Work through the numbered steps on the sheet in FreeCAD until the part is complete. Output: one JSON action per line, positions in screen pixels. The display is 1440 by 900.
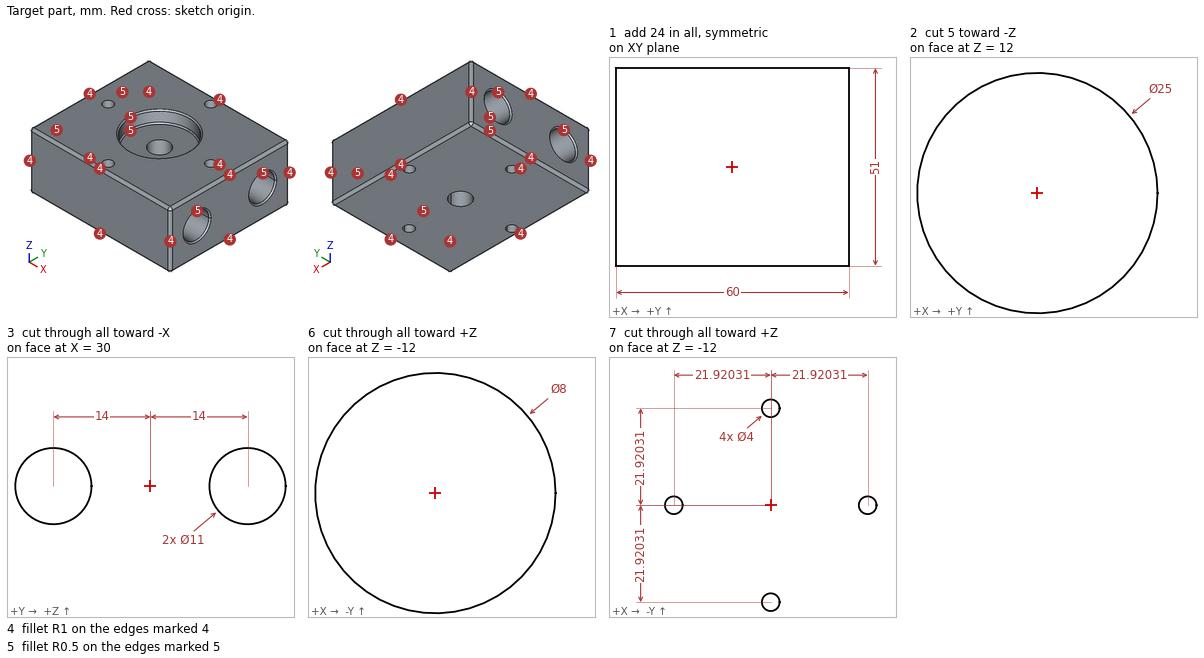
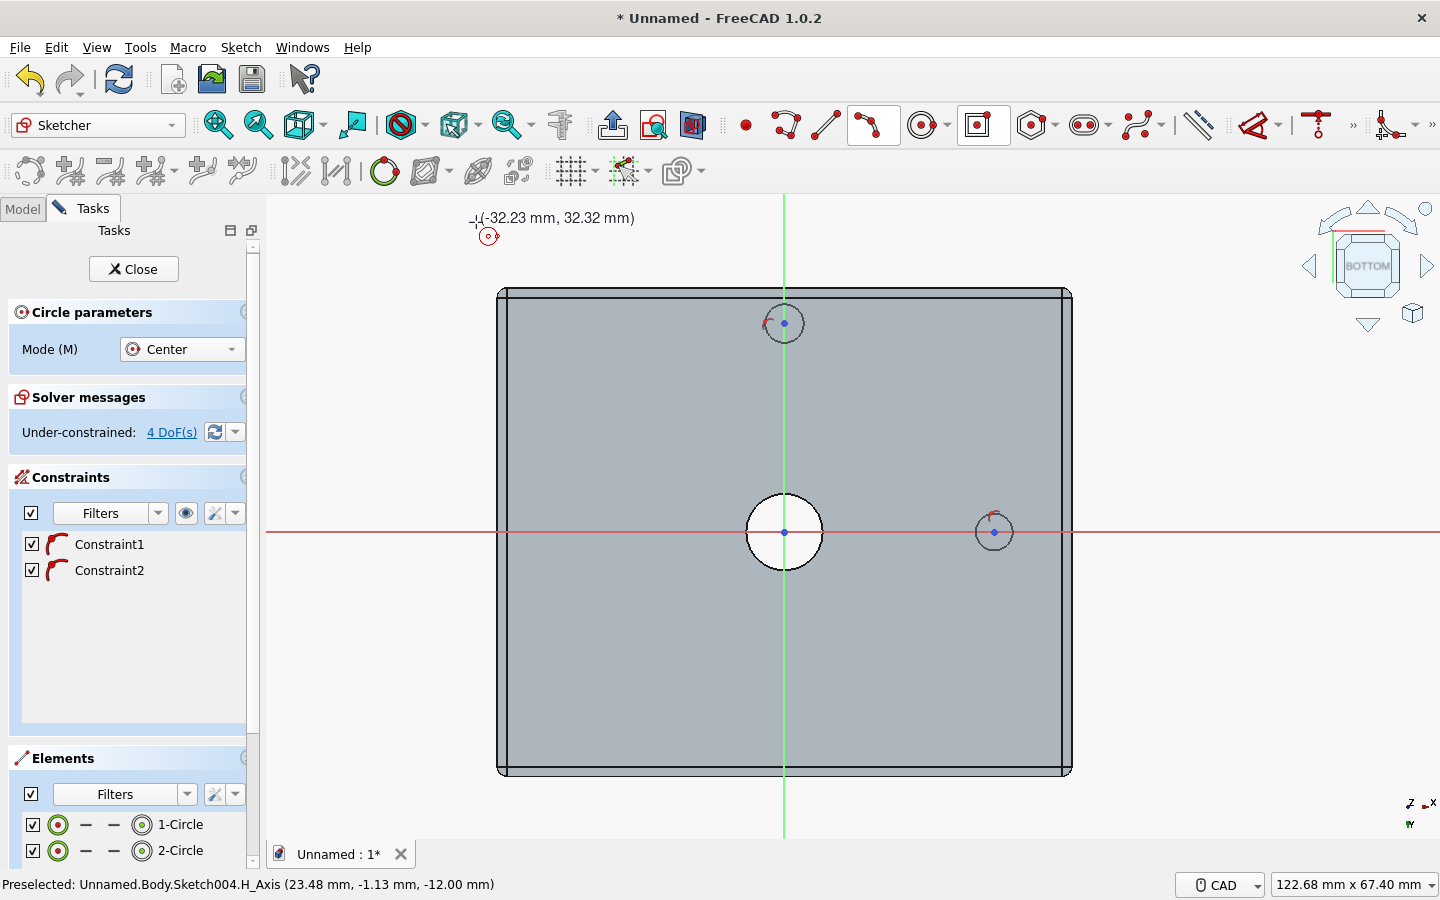
{"action": "left_click", "coordinate": [784, 742]}
{"action": "left_click", "coordinate": [802, 735]}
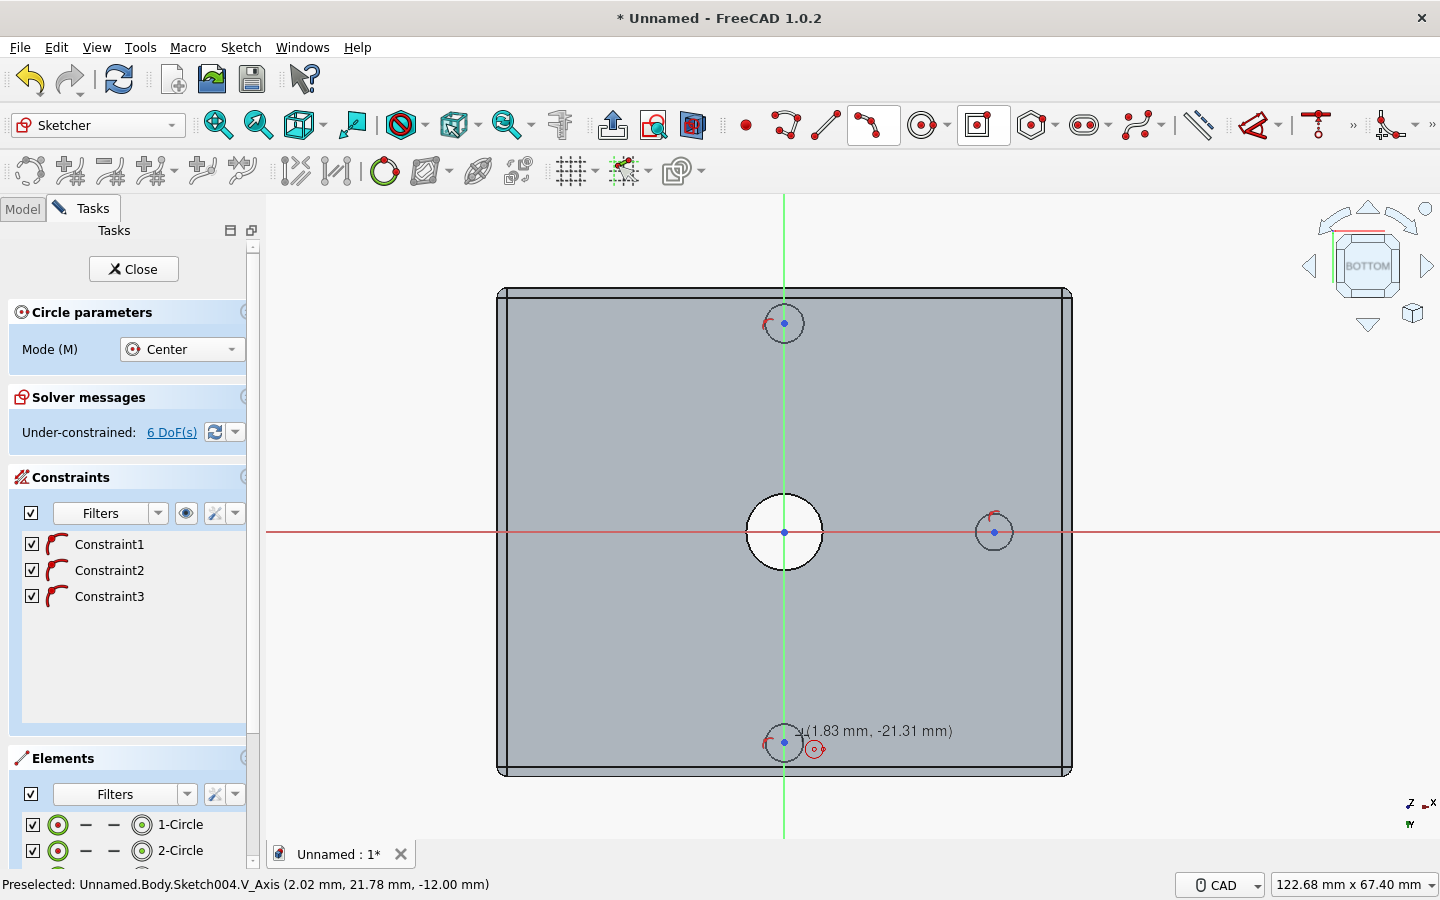
{"action": "left_click", "coordinate": [575, 532]}
{"action": "left_click", "coordinate": [581, 514]}
{"action": "key", "text": "Escape"}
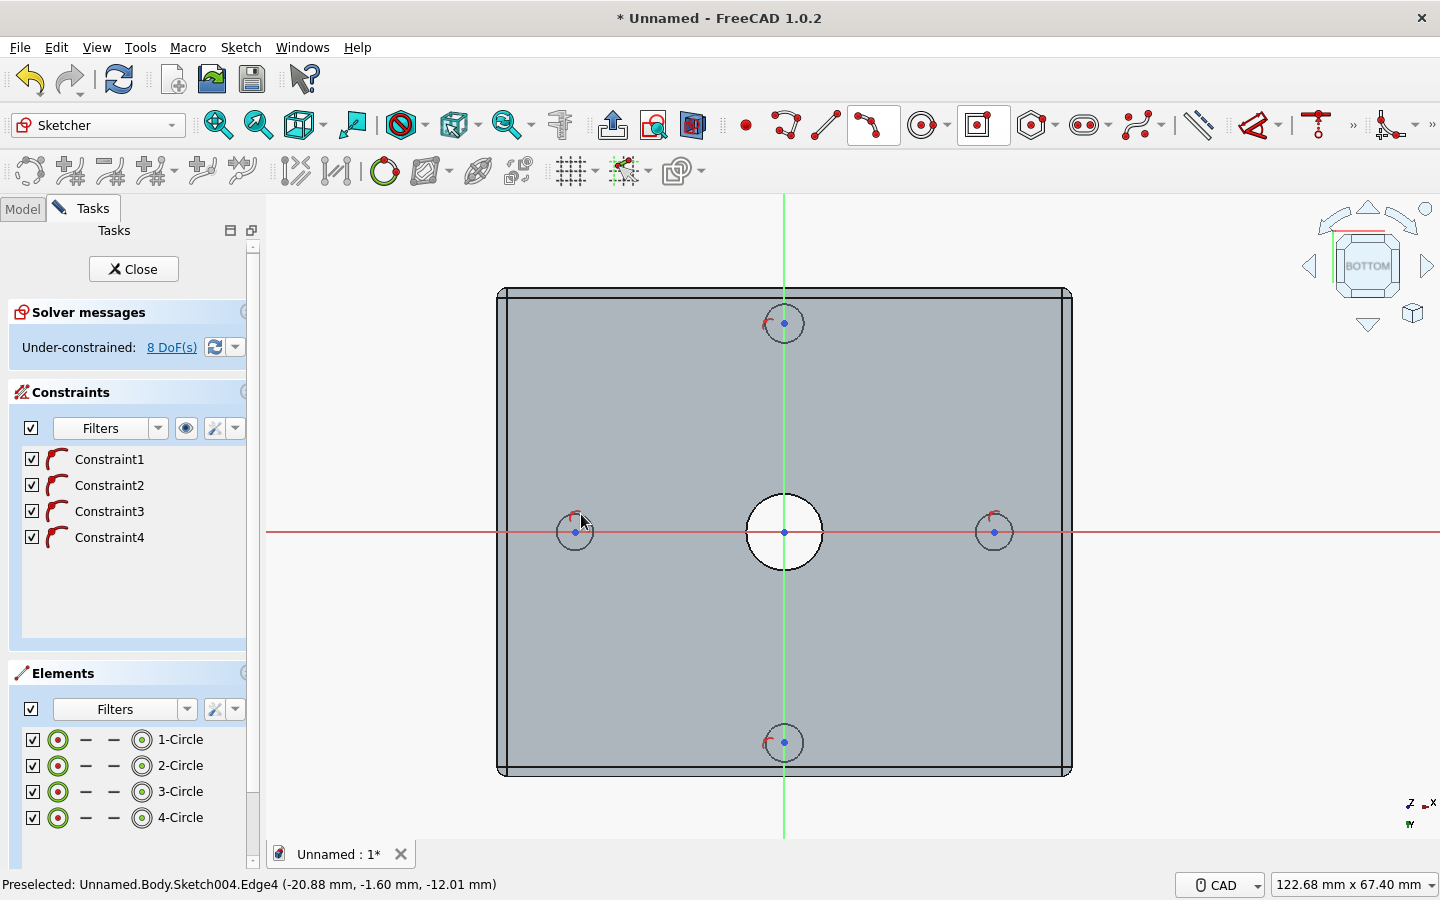
{"action": "left_click", "coordinate": [798, 310]}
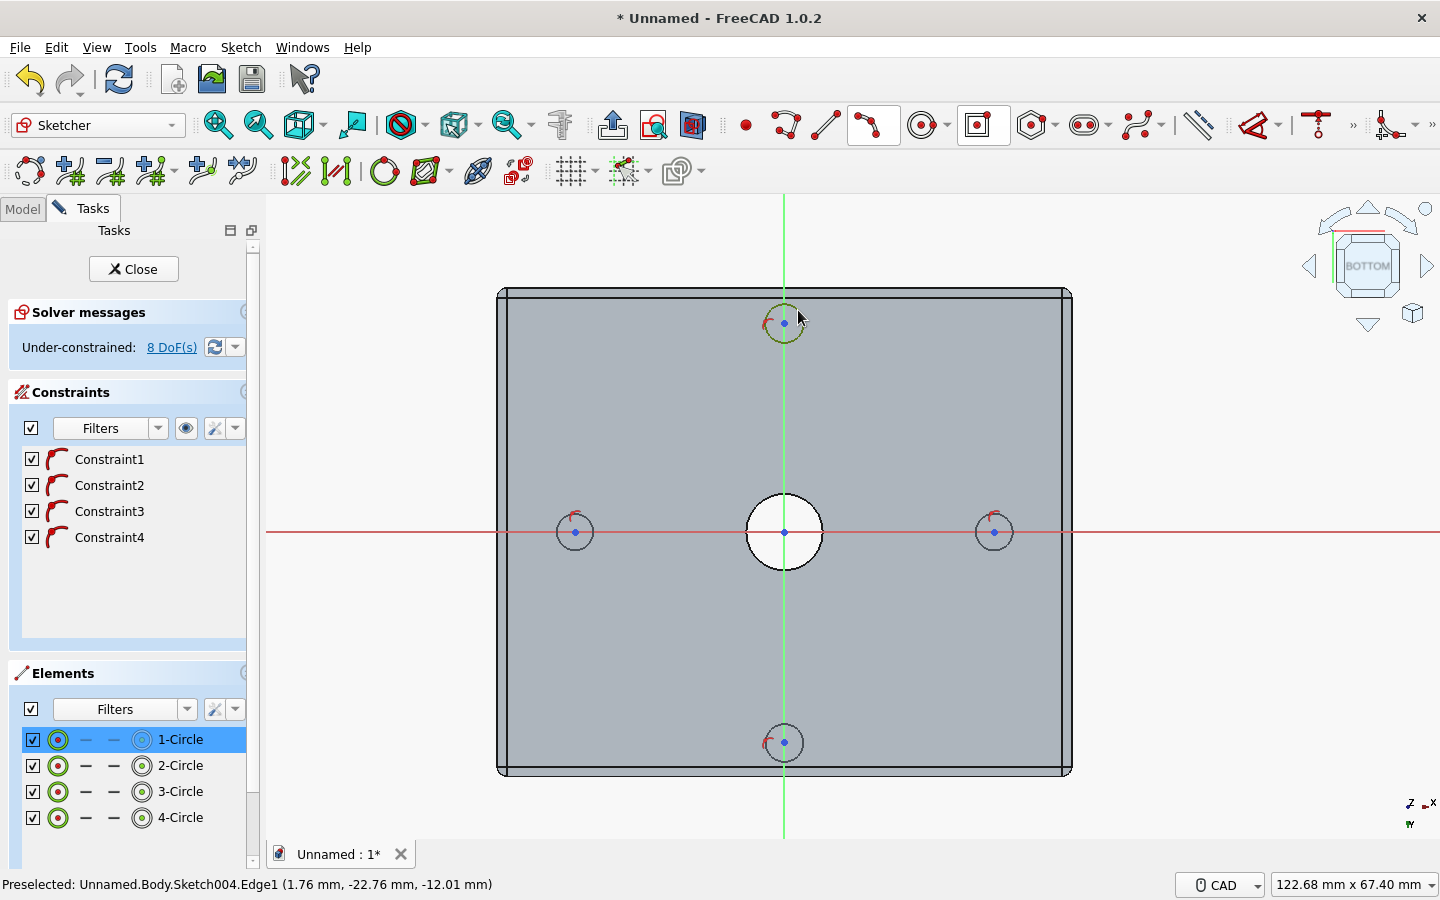
{"action": "left_click", "coordinate": [1007, 519]}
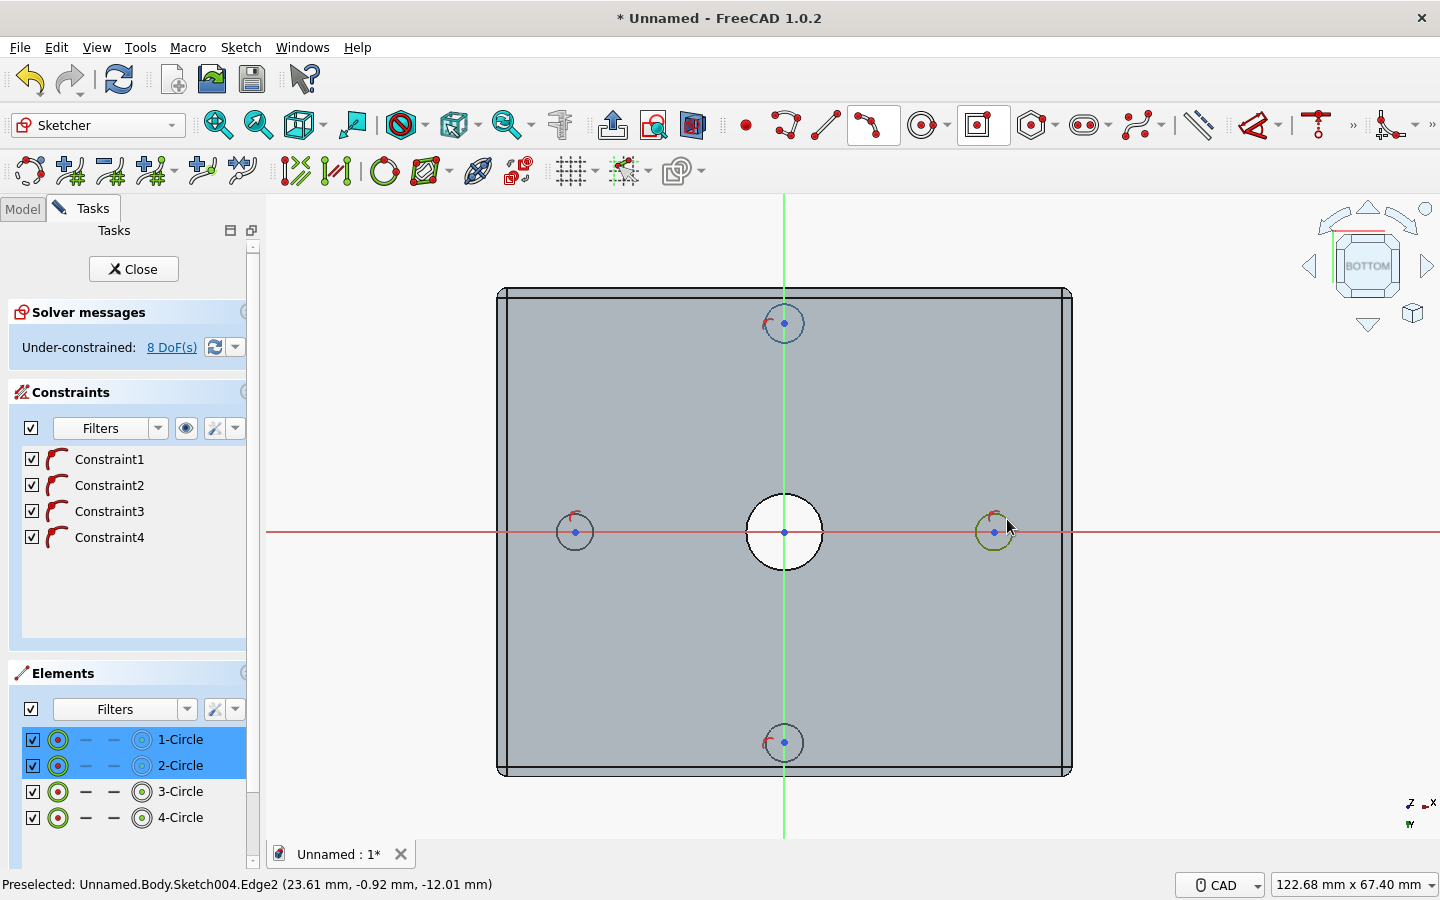
{"action": "left_click", "coordinate": [798, 730]}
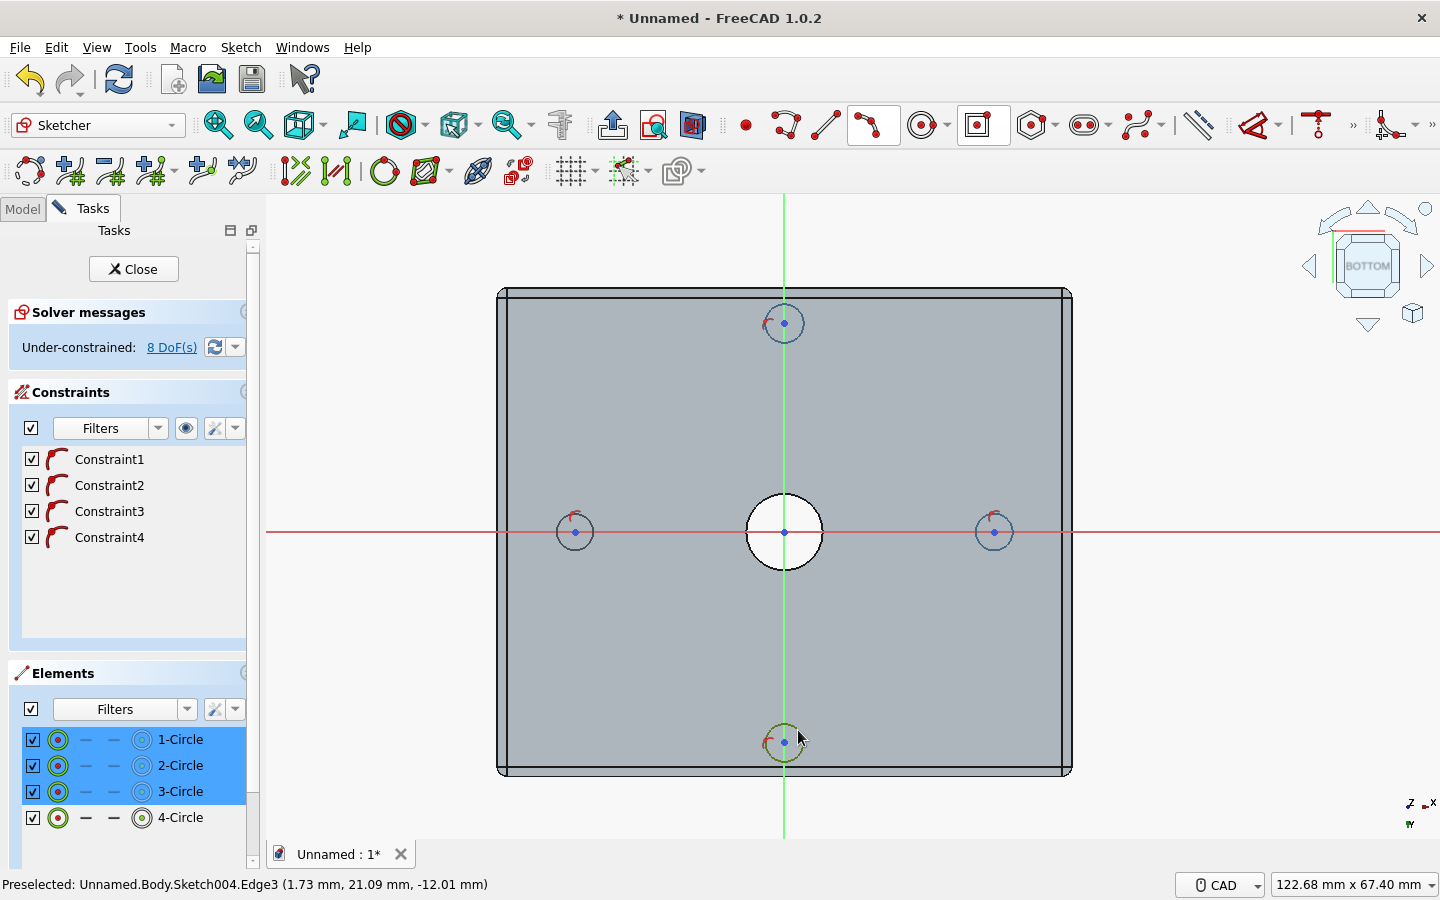
{"action": "left_click", "coordinate": [588, 519]}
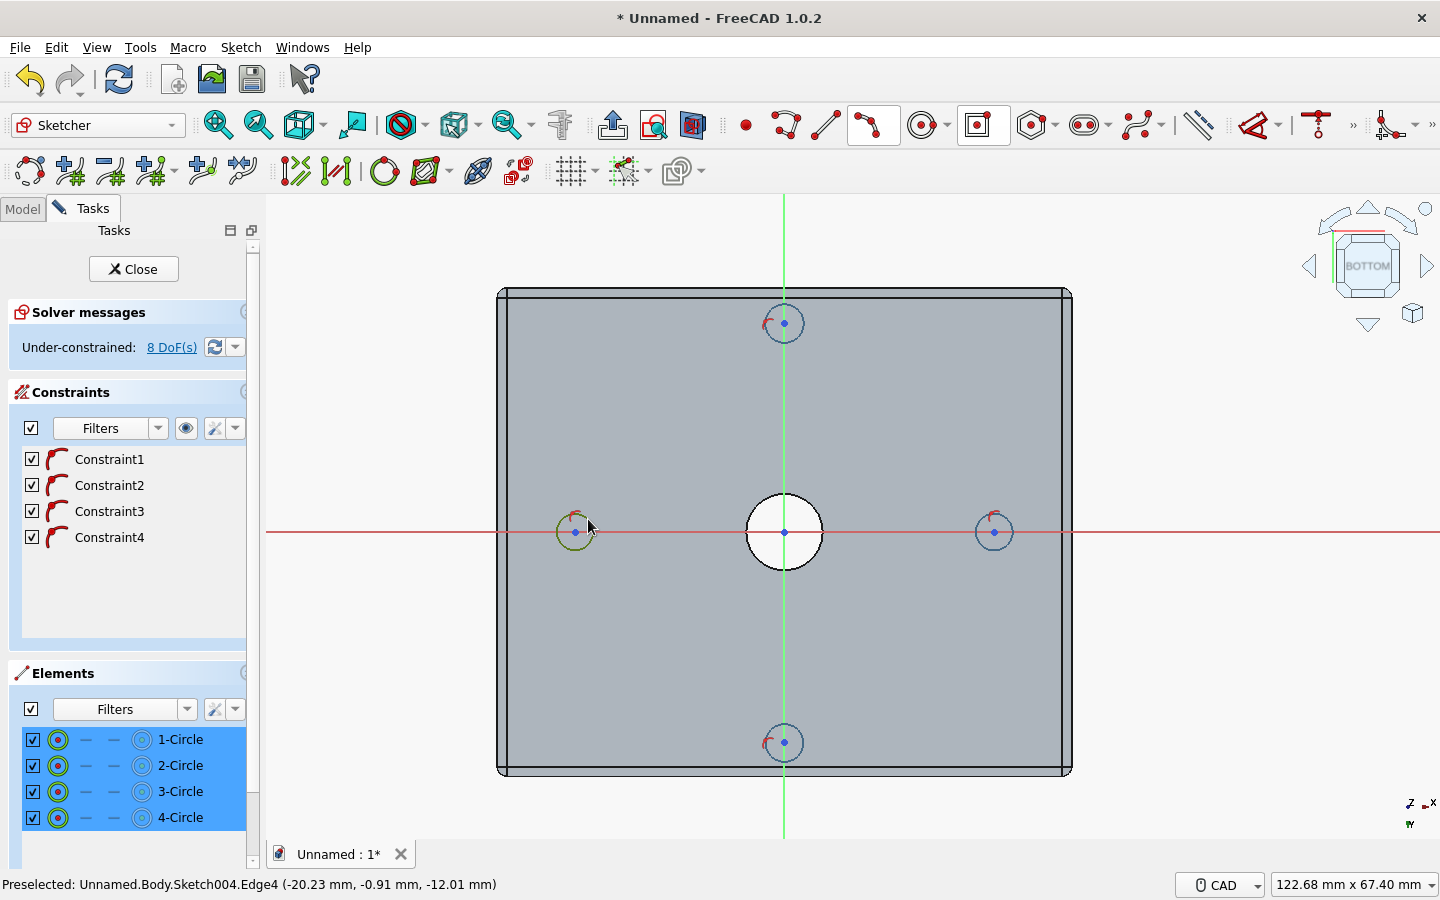
{"action": "key", "text": "e"}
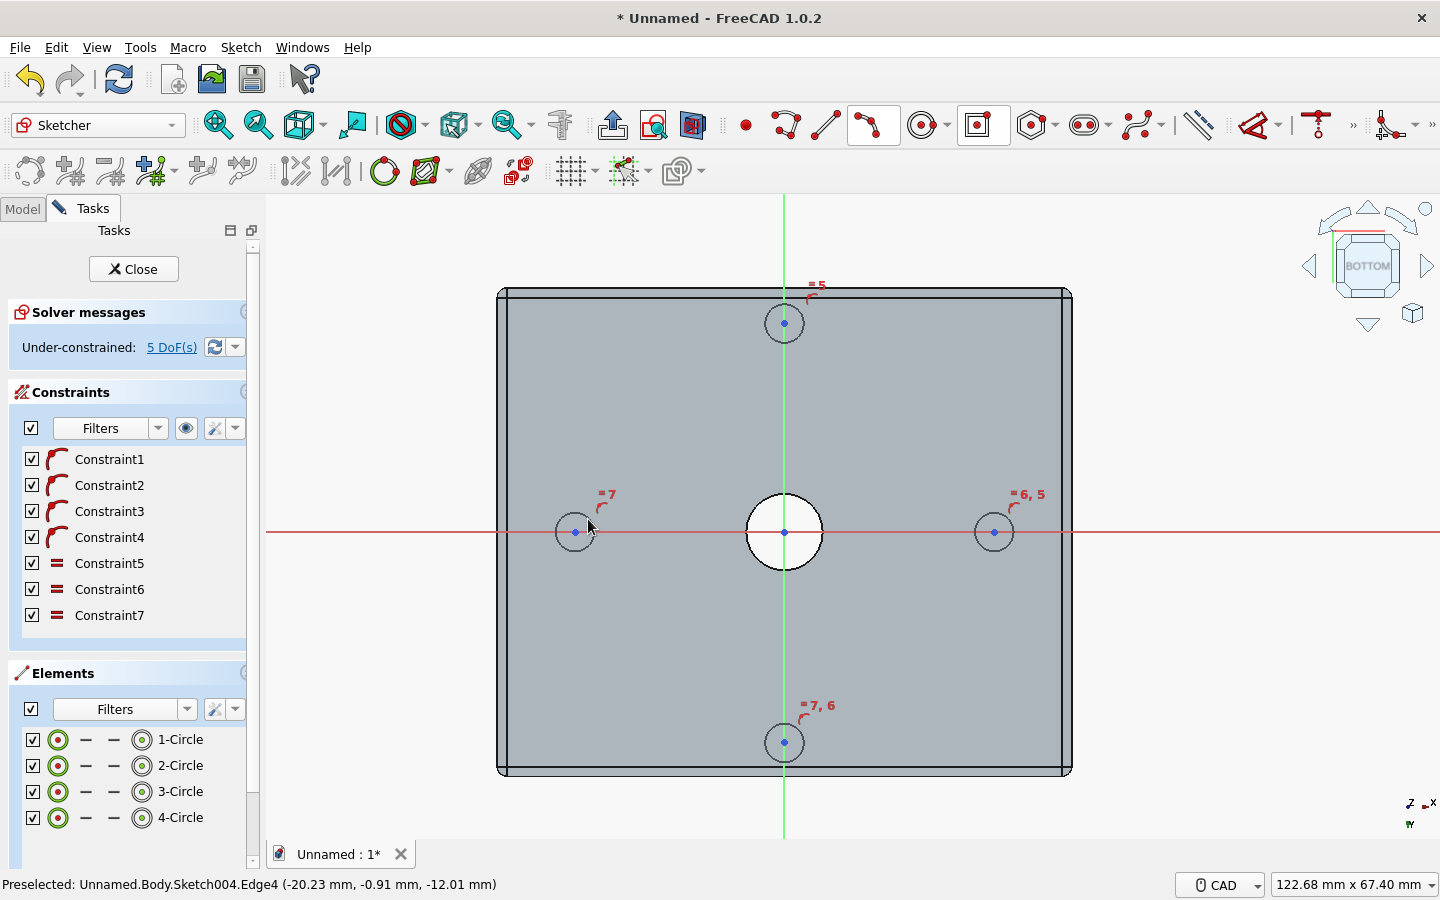
{"action": "left_click", "coordinate": [1254, 126]}